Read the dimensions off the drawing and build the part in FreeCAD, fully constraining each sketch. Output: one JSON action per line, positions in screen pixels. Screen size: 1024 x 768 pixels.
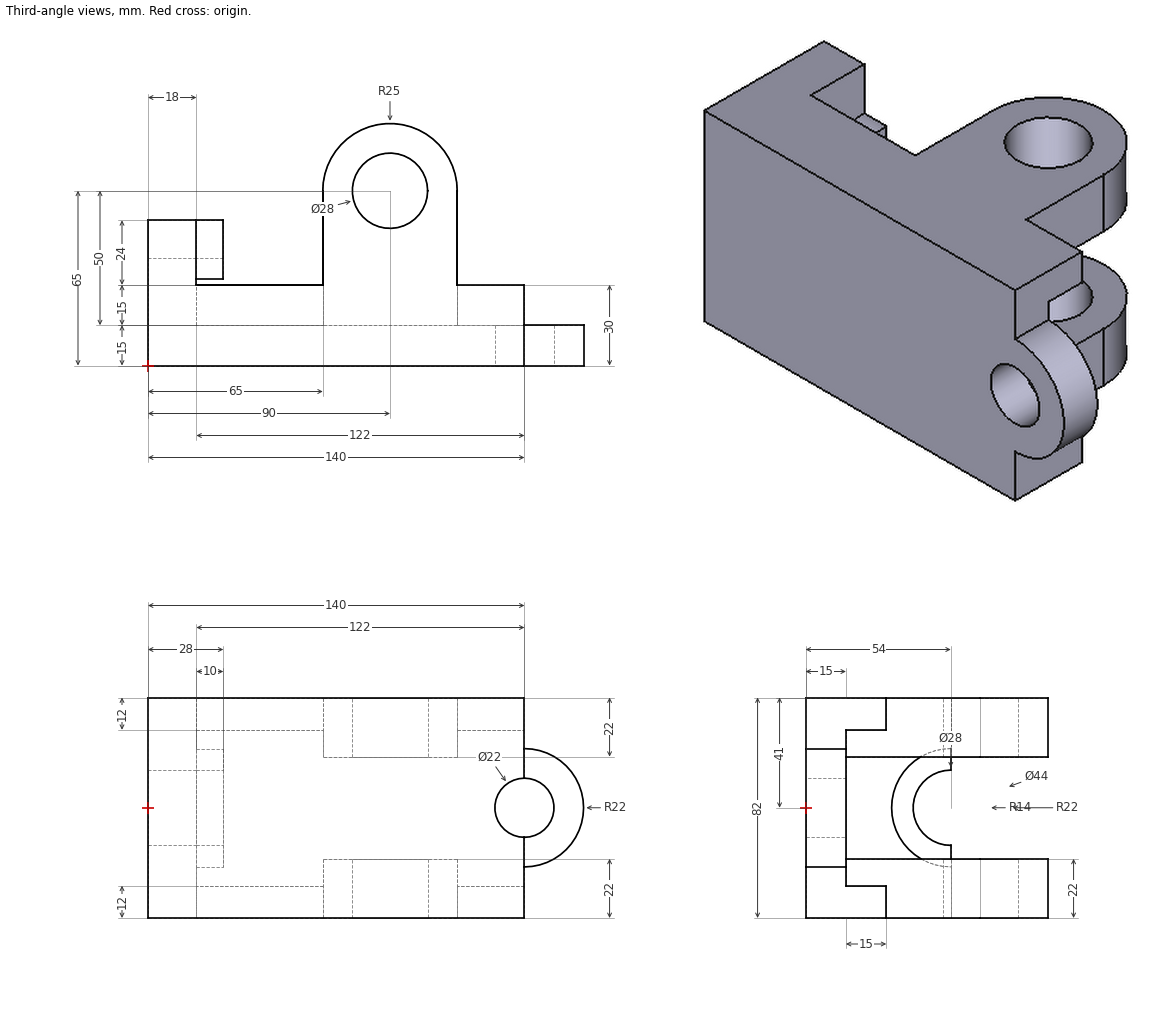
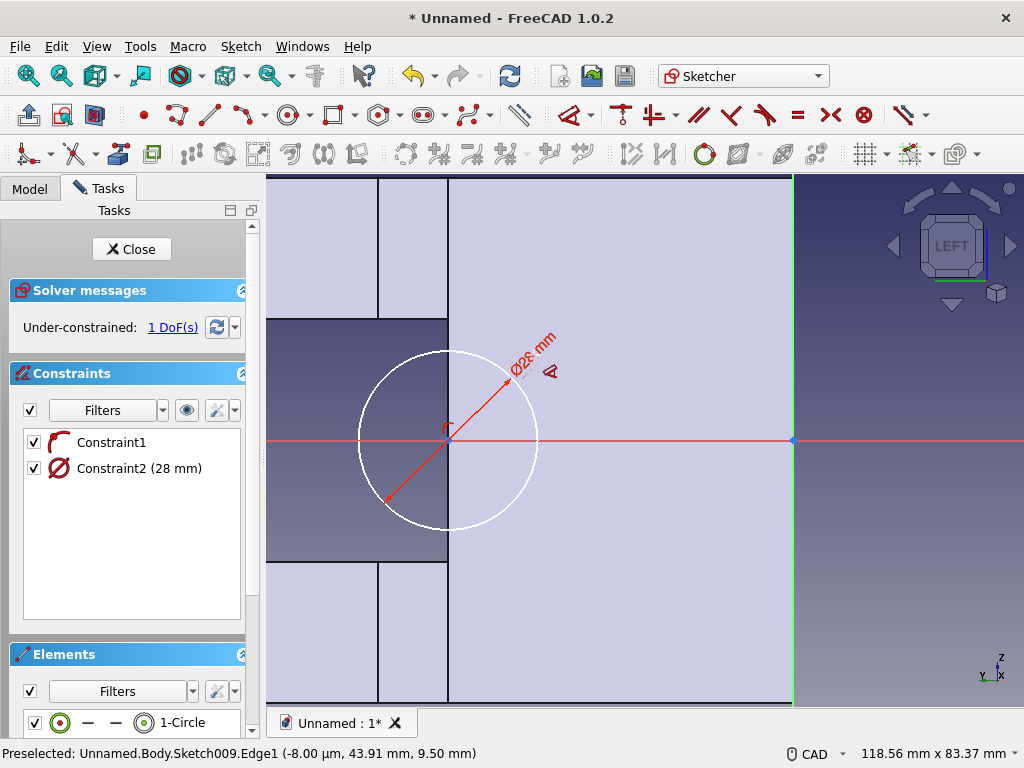
{"action": "left_click", "coordinate": [448, 440]}
{"action": "left_click", "coordinate": [621, 474]}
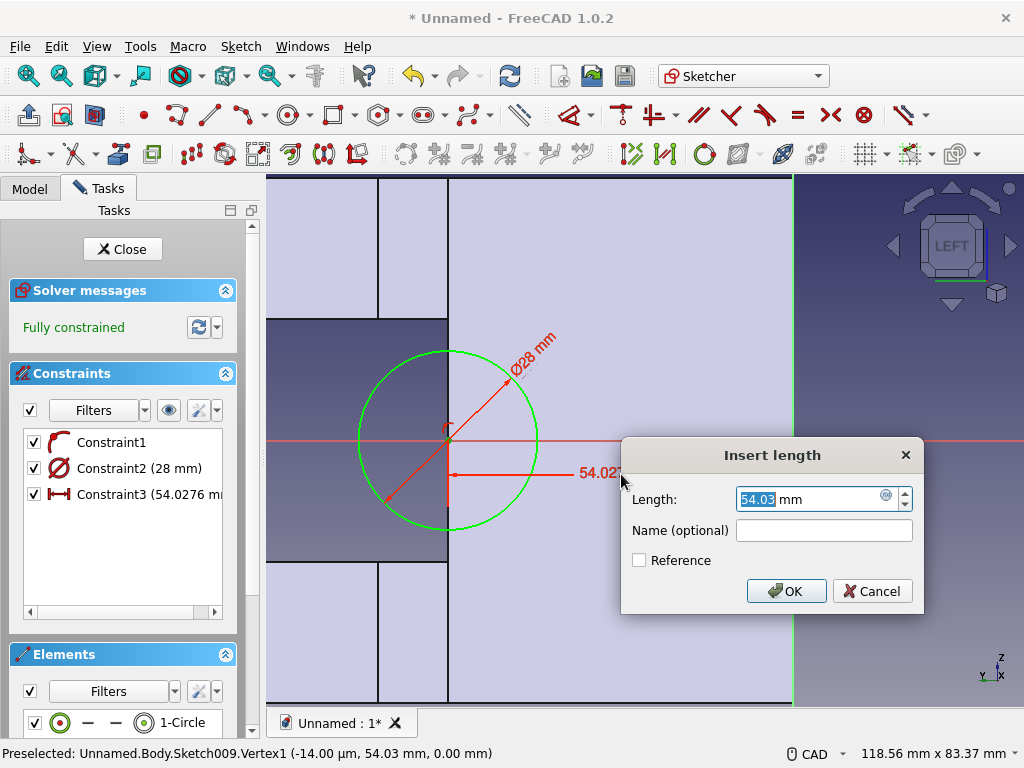
{"action": "type", "text": "54"}
{"action": "key", "text": "Return"}
{"action": "key", "text": "Escape"}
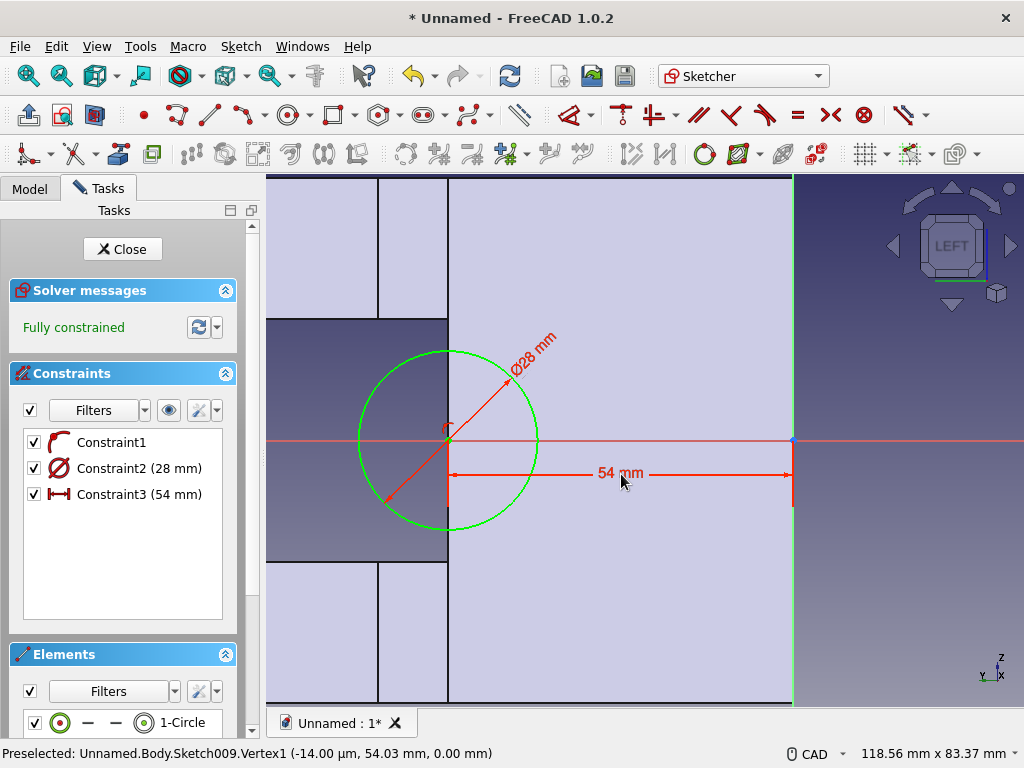
{"action": "left_click", "coordinate": [123, 249]}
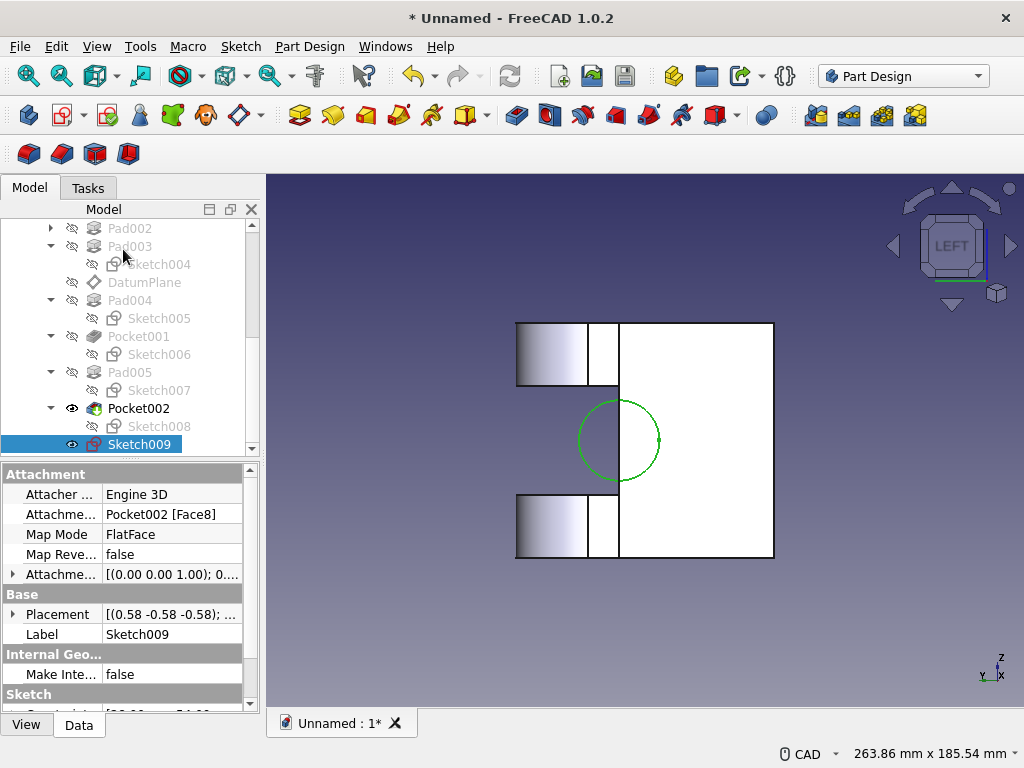
{"action": "left_click", "coordinate": [517, 116]}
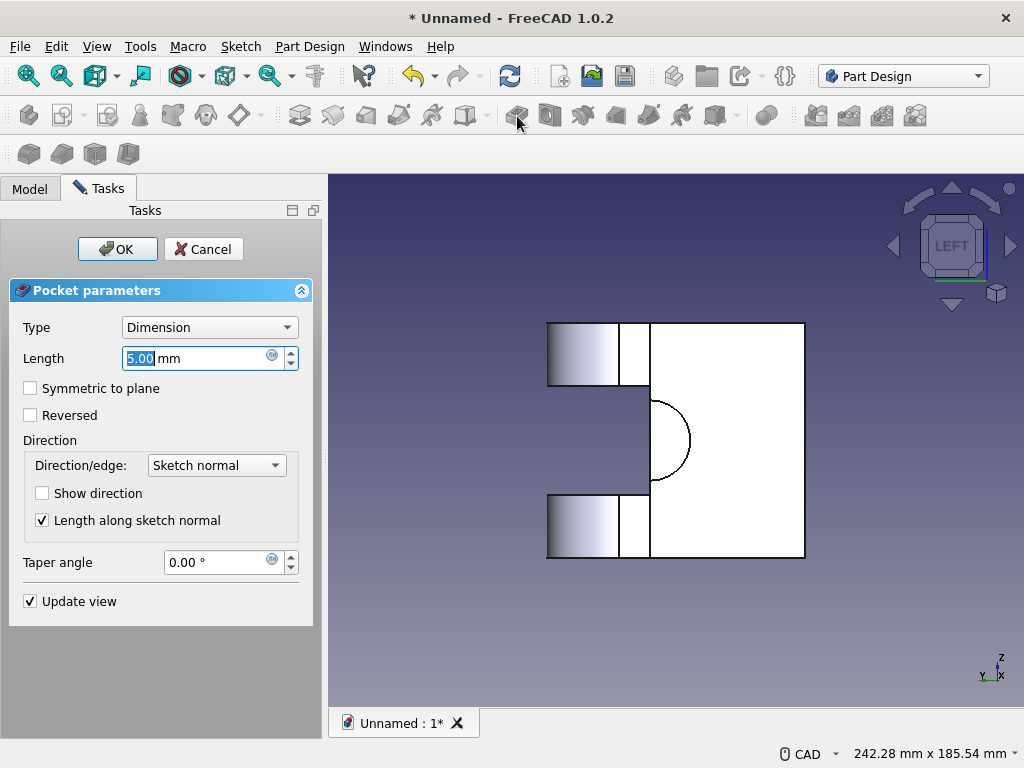
{"action": "type", "text": "28"}
{"action": "key", "text": "Tab"}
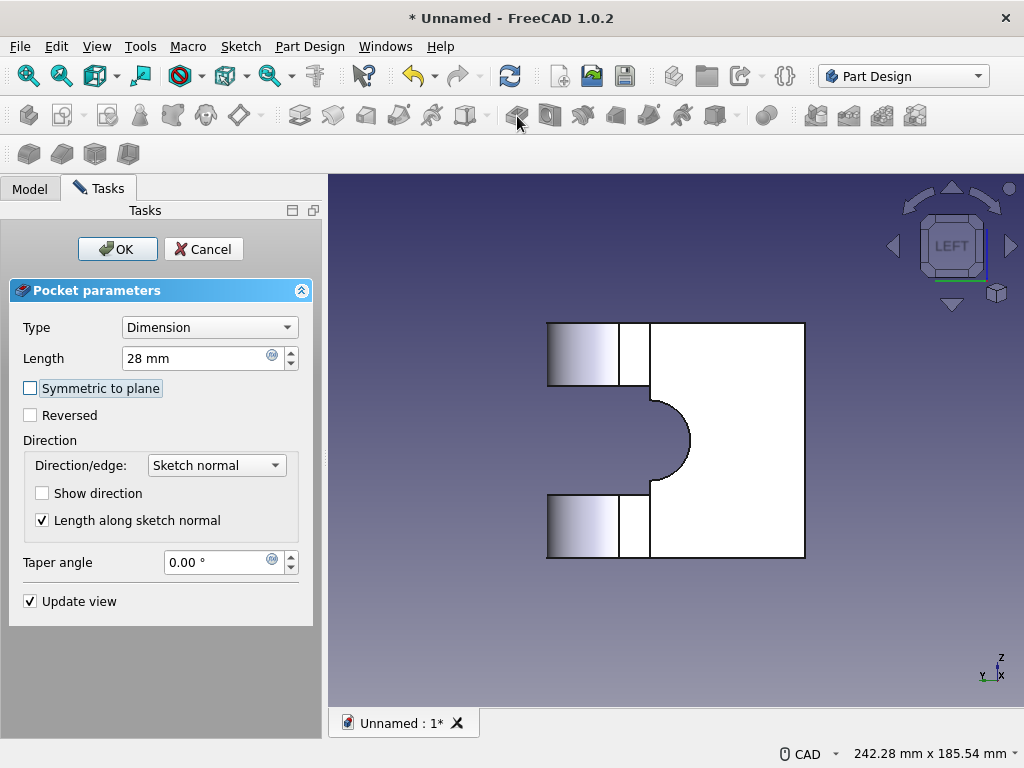
{"action": "left_click", "coordinate": [118, 249]}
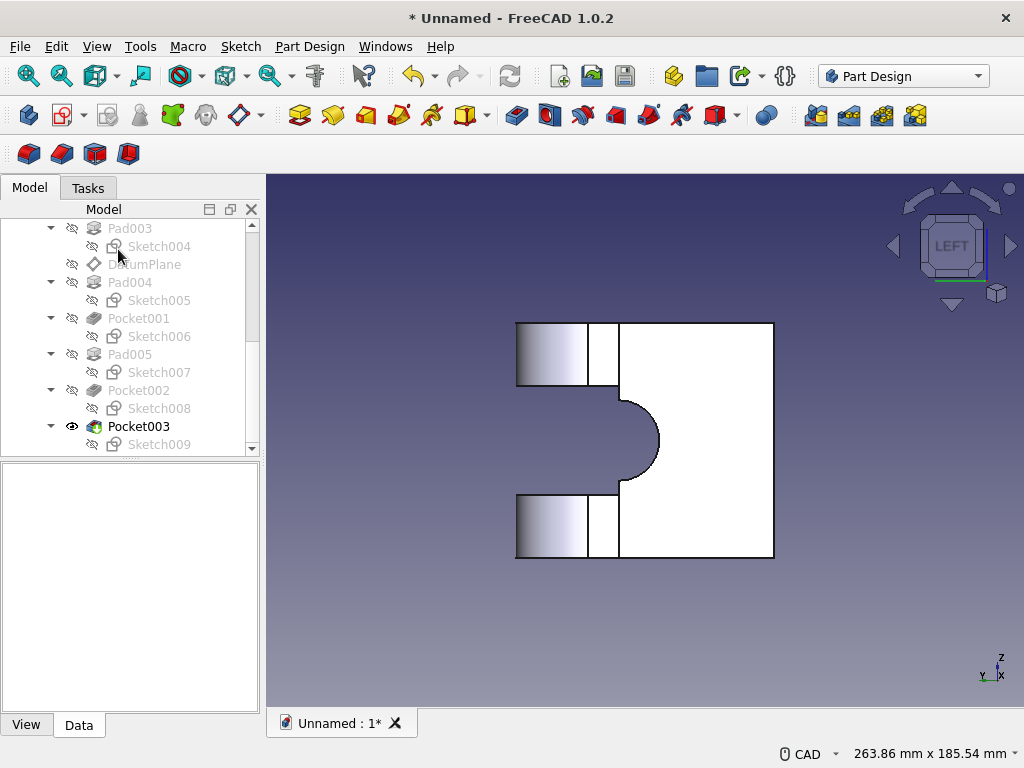
{"action": "key", "text": "v f"}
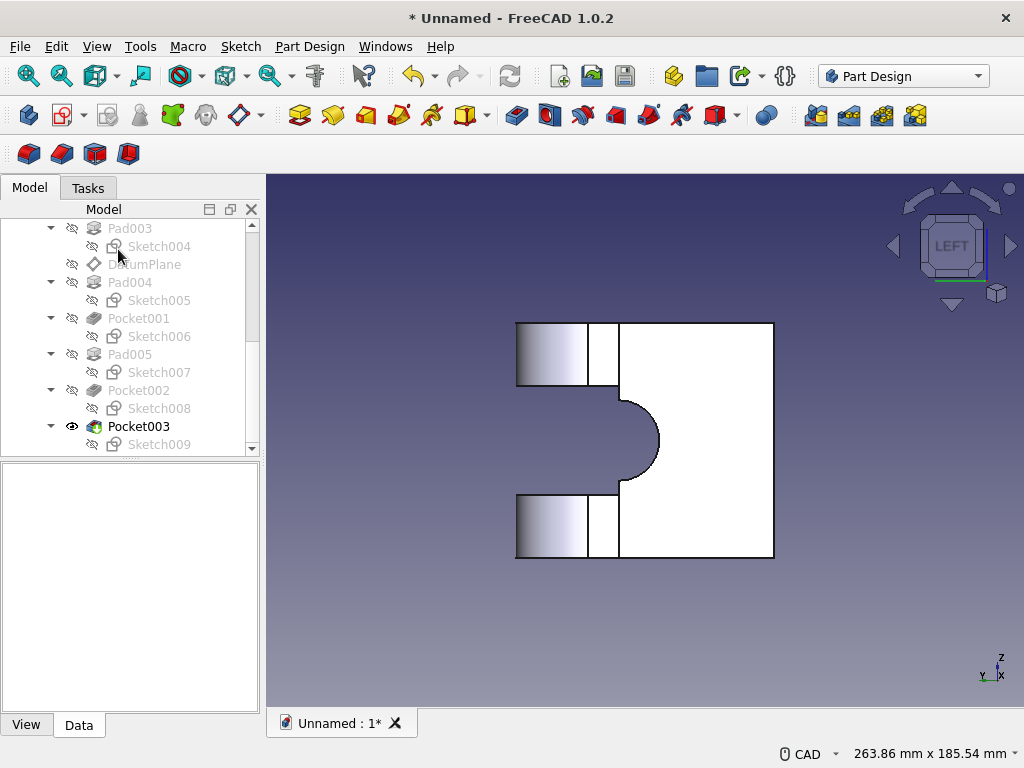
{"action": "key", "text": "0"}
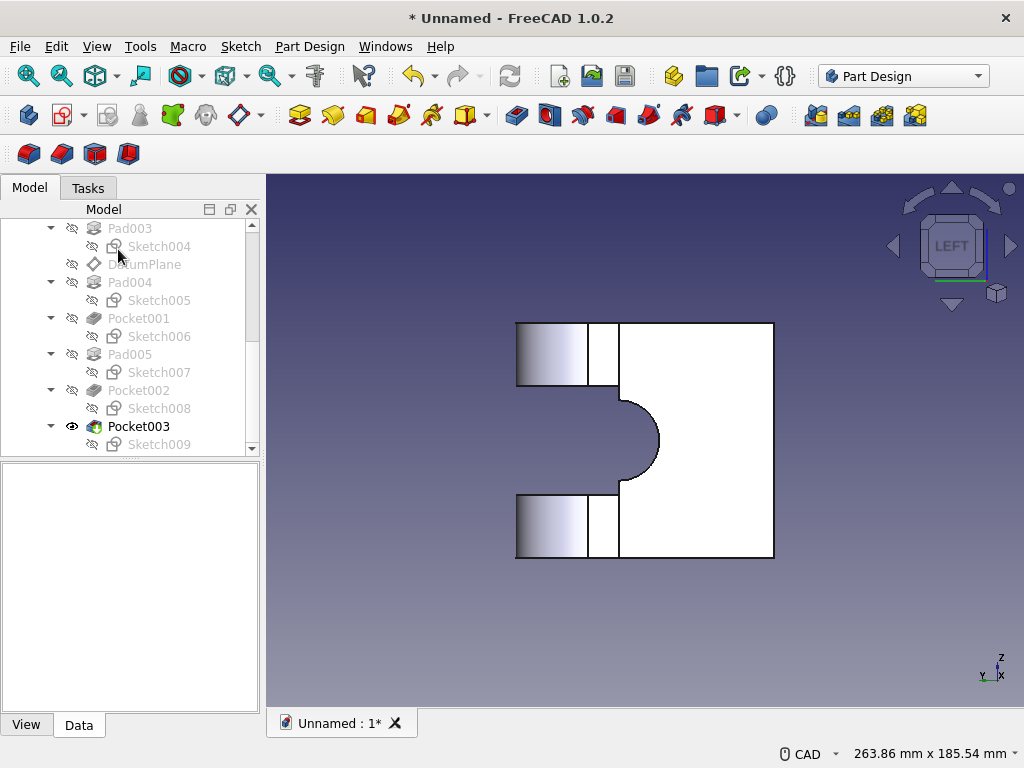
{"action": "left_click", "coordinate": [594, 516]}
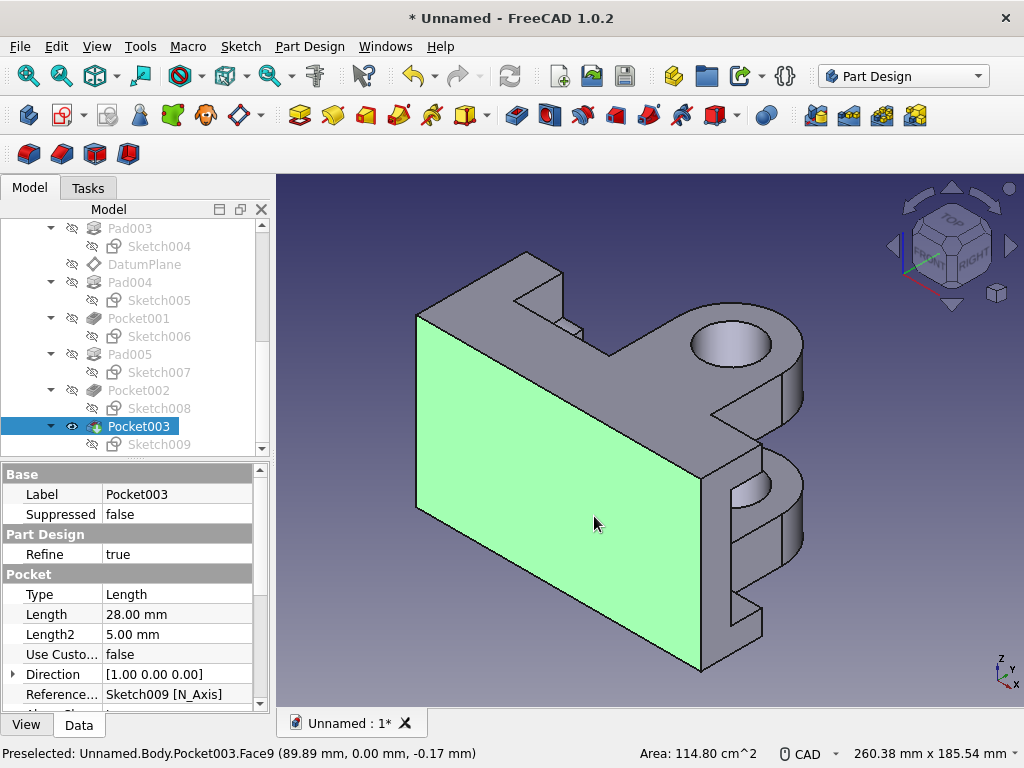
{"action": "left_click", "coordinate": [62, 116]}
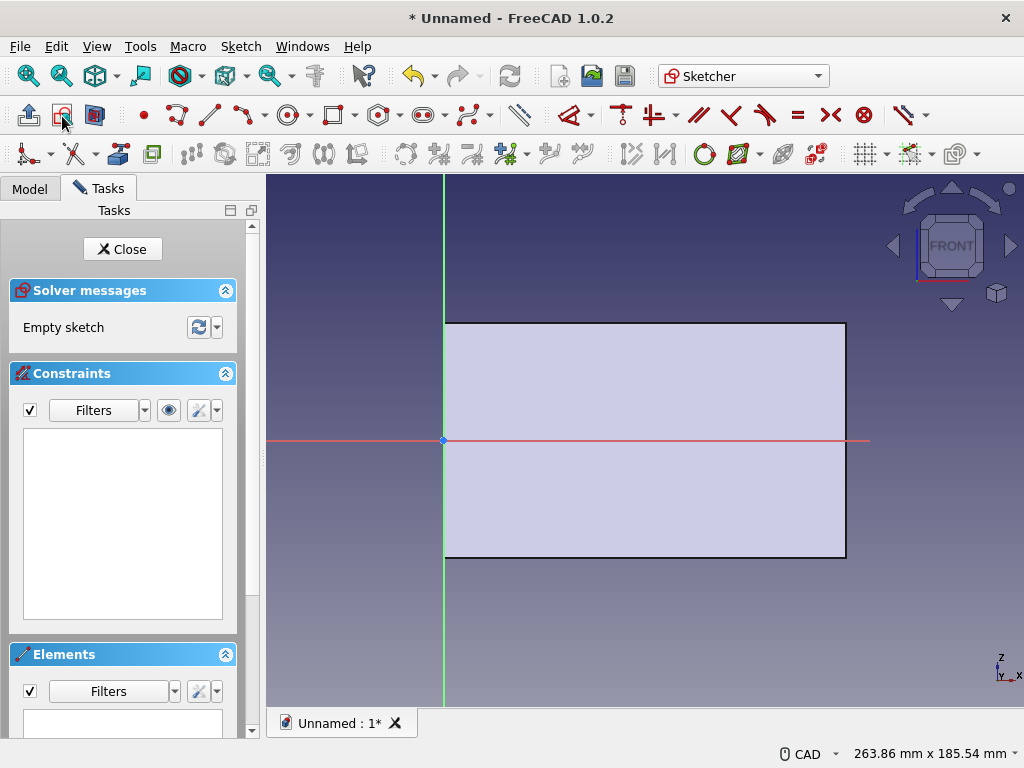
{"action": "scroll", "coordinate": [576, 440], "scroll_direction": "down", "scroll_amount": 5}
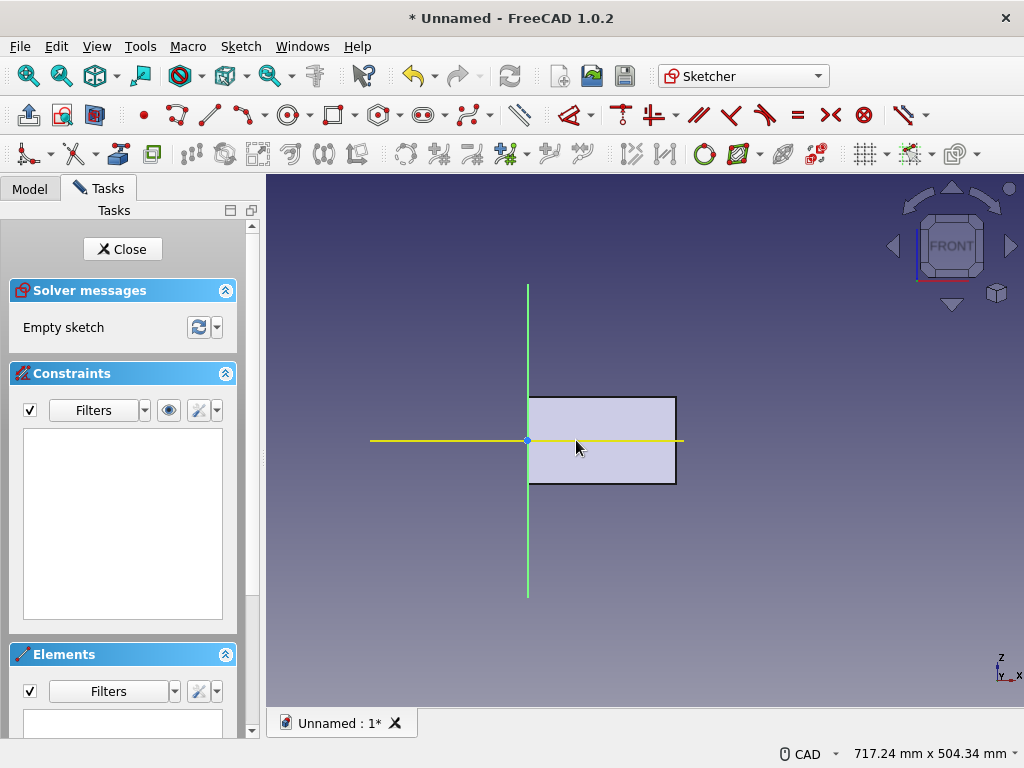
{"action": "scroll", "coordinate": [705, 440], "scroll_direction": "up", "scroll_amount": 10}